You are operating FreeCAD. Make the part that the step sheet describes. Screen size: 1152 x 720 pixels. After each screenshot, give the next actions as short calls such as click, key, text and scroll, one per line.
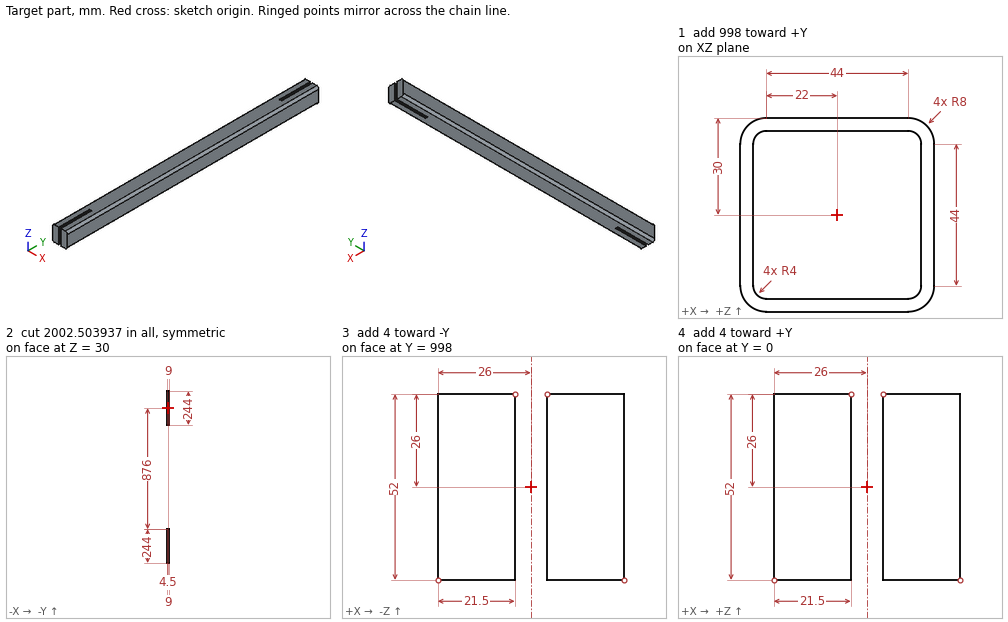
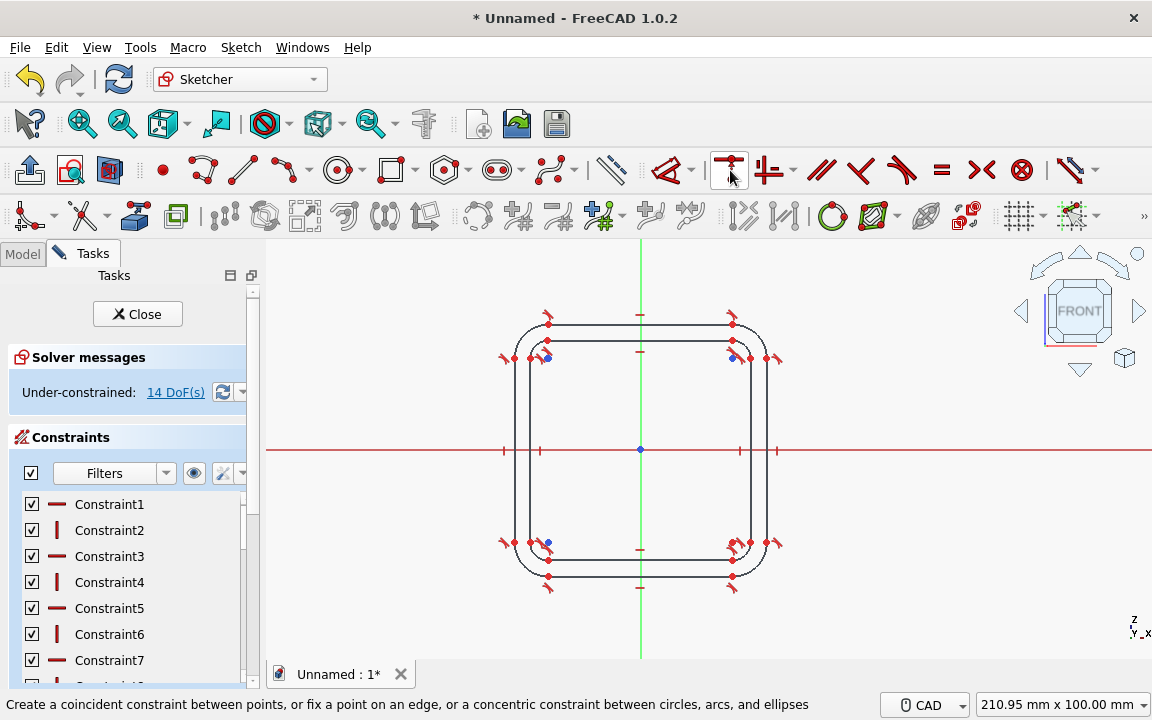
click(763, 343)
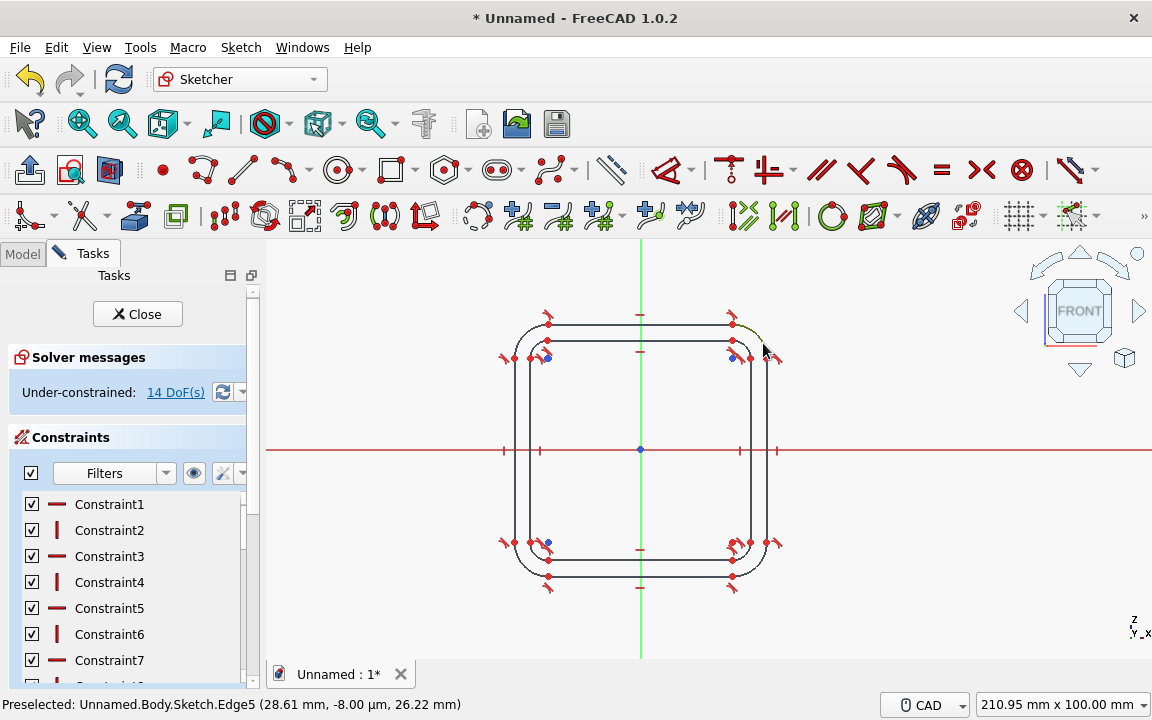
click(745, 346)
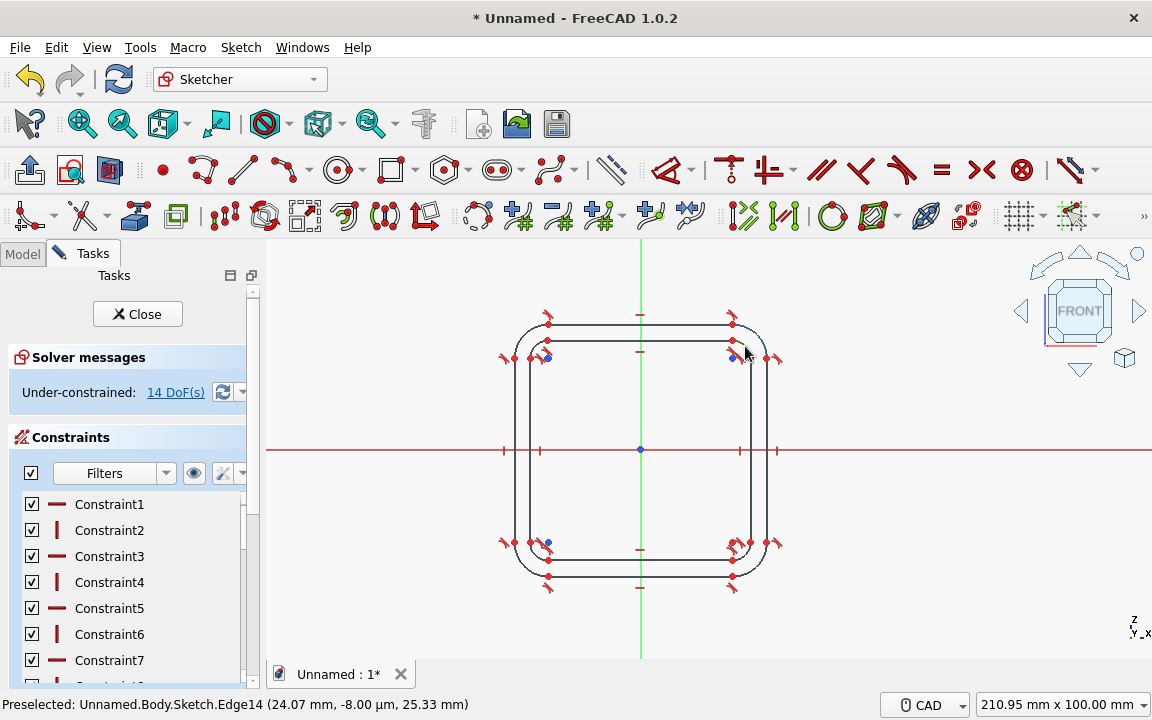
click(730, 170)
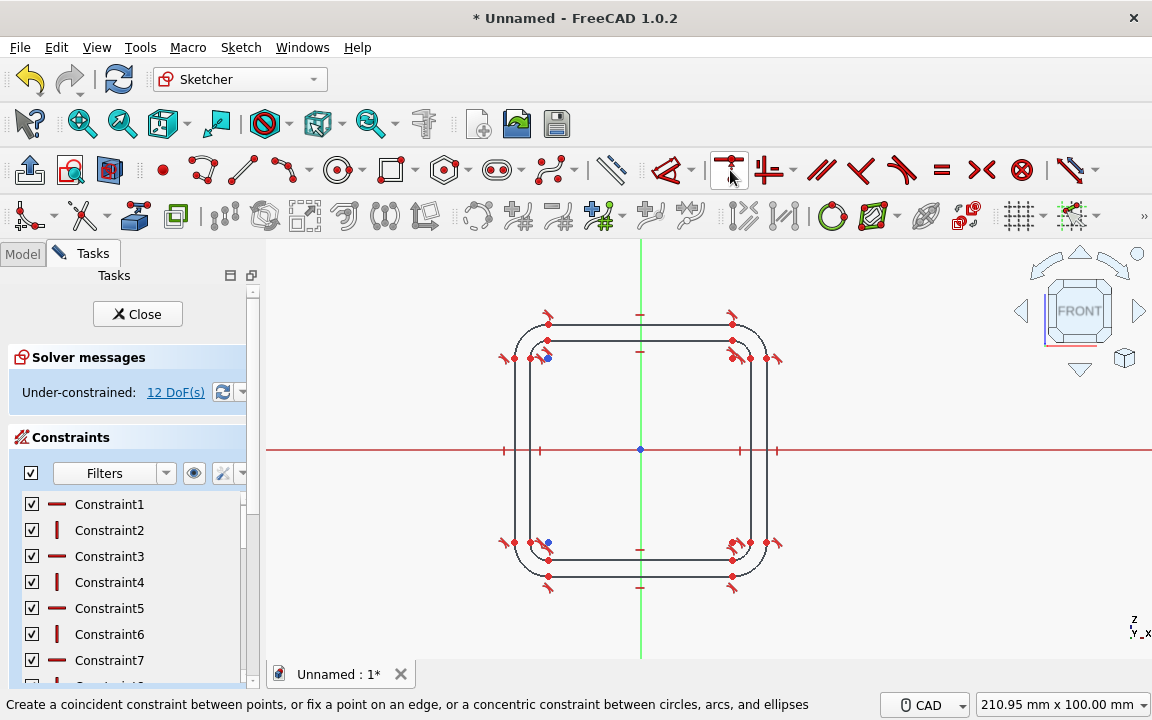
click(533, 328)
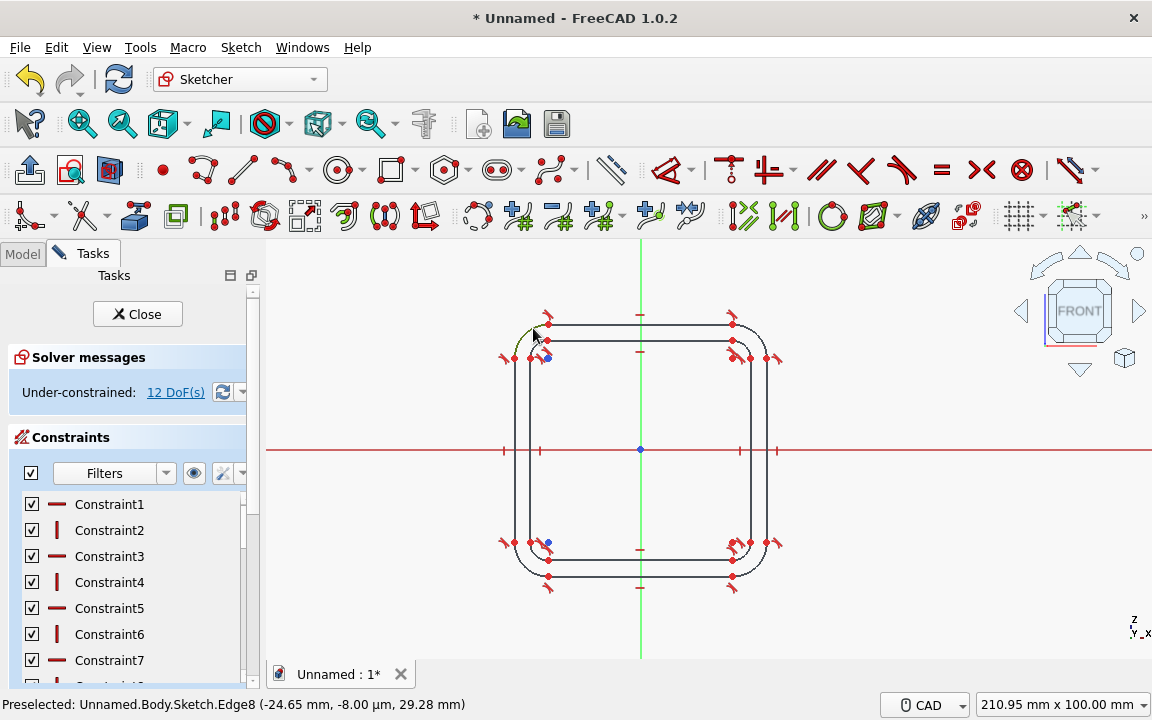
click(535, 346)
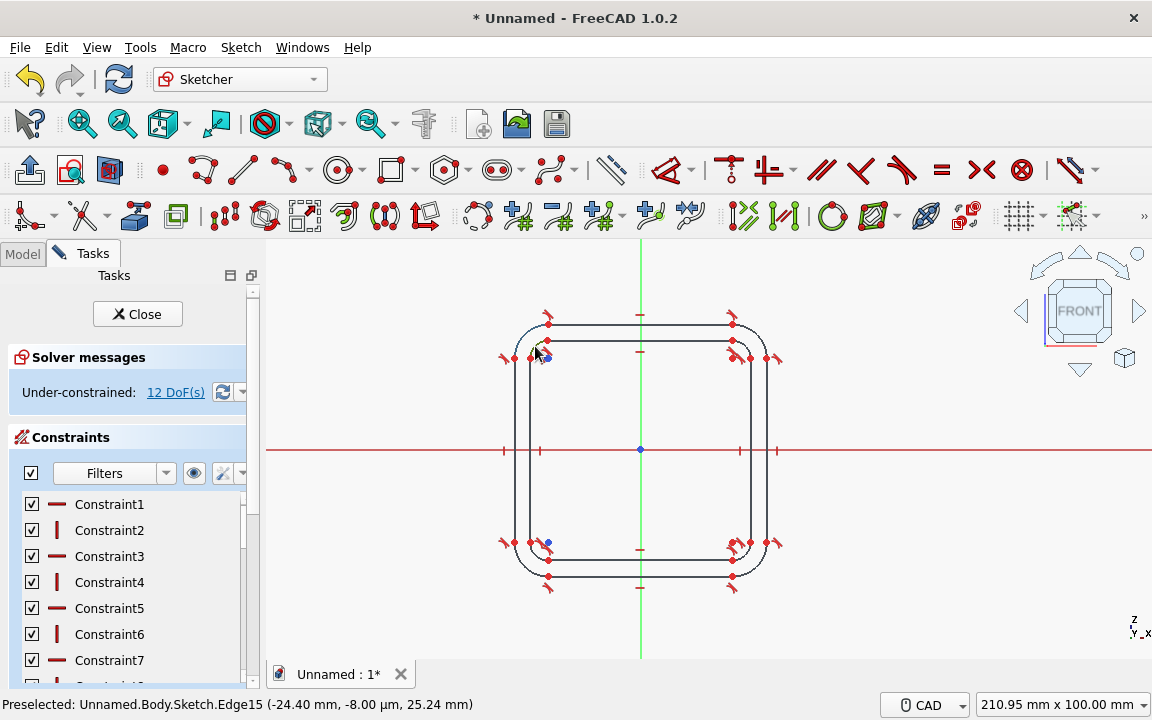
click(730, 170)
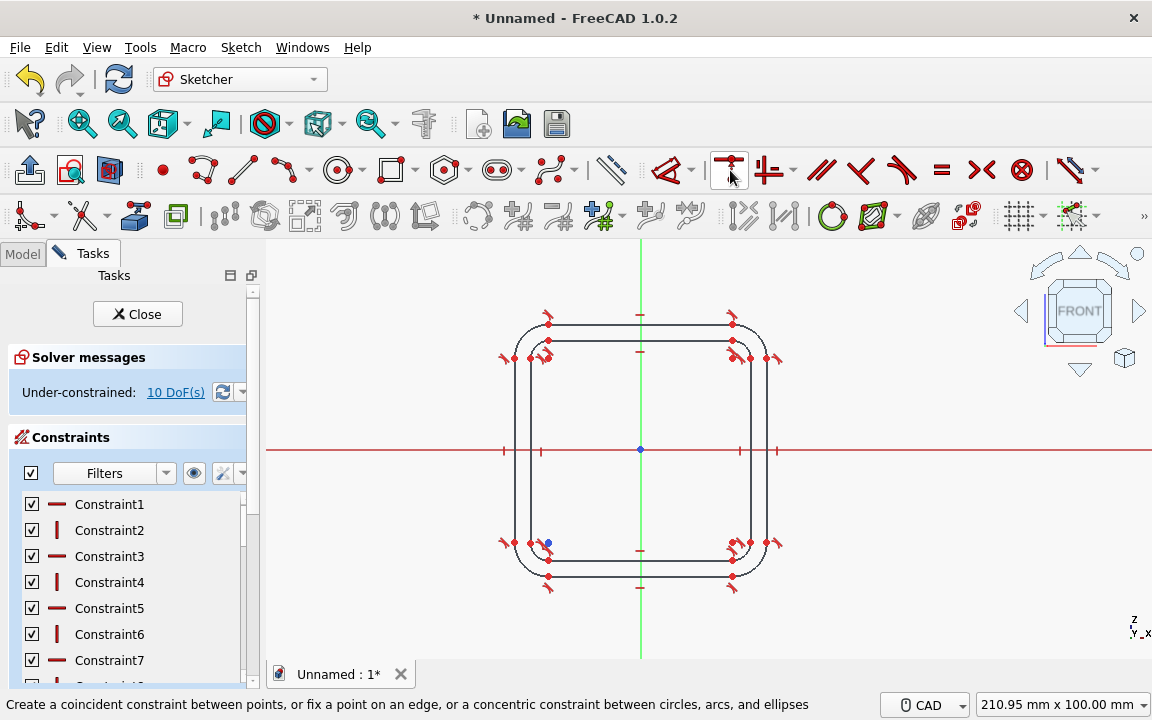
click(763, 343)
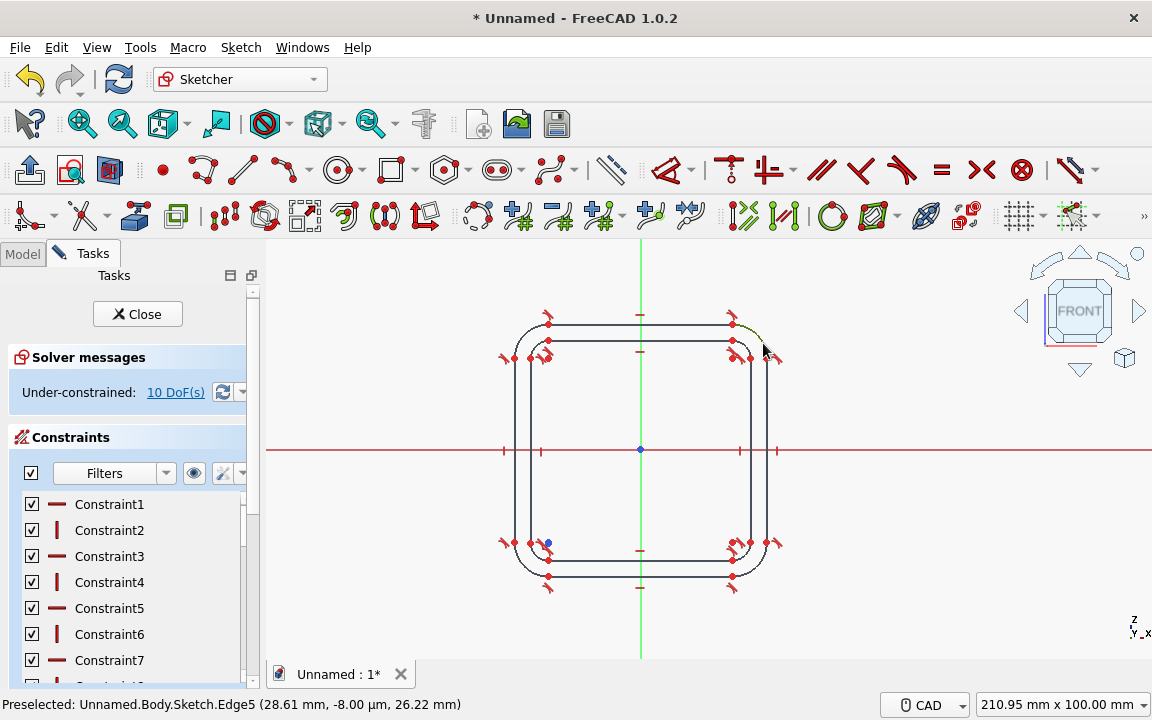
click(748, 573)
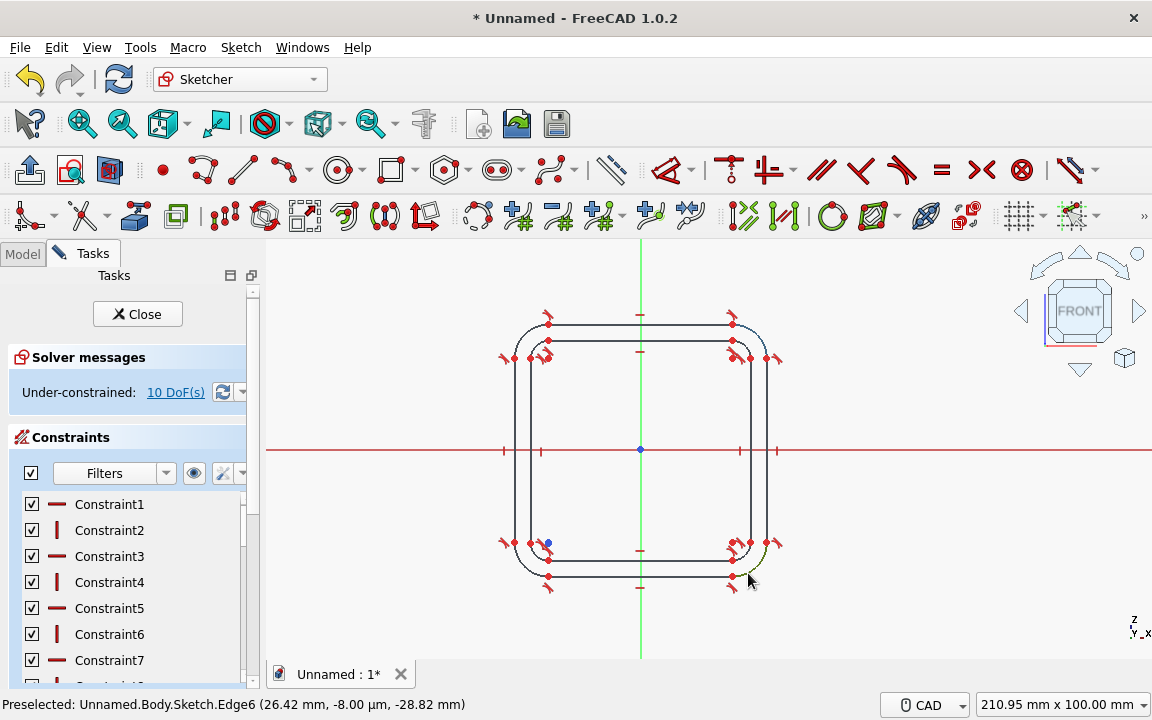
click(518, 558)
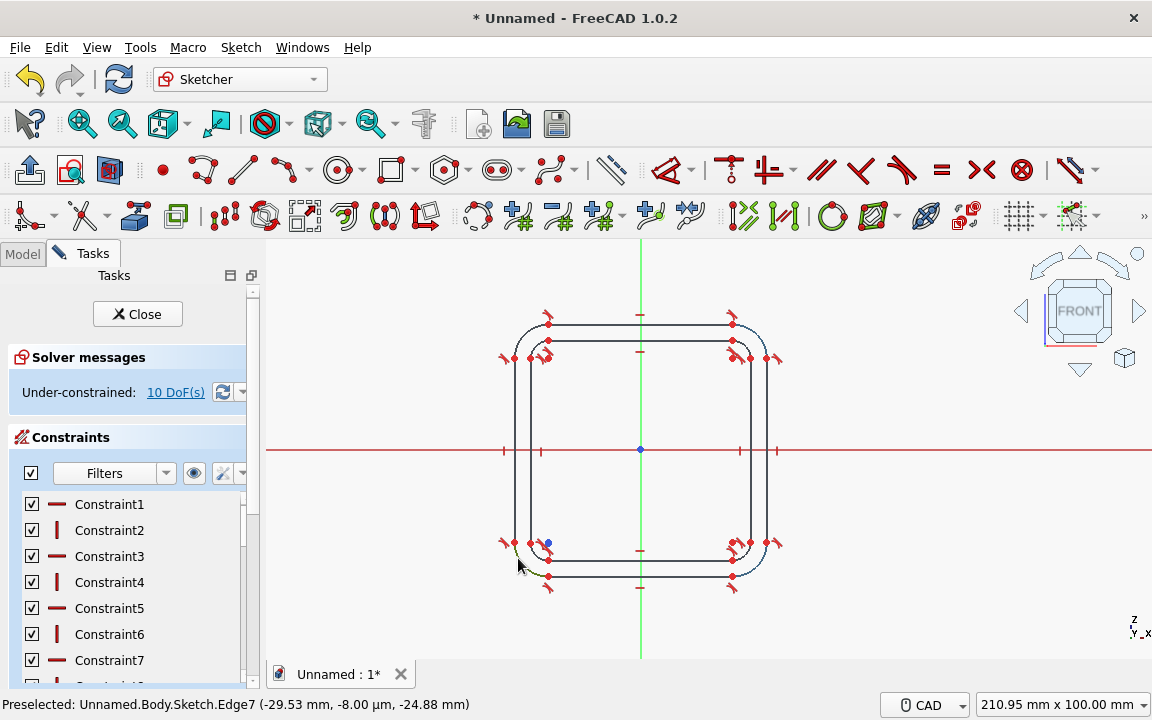
click(533, 328)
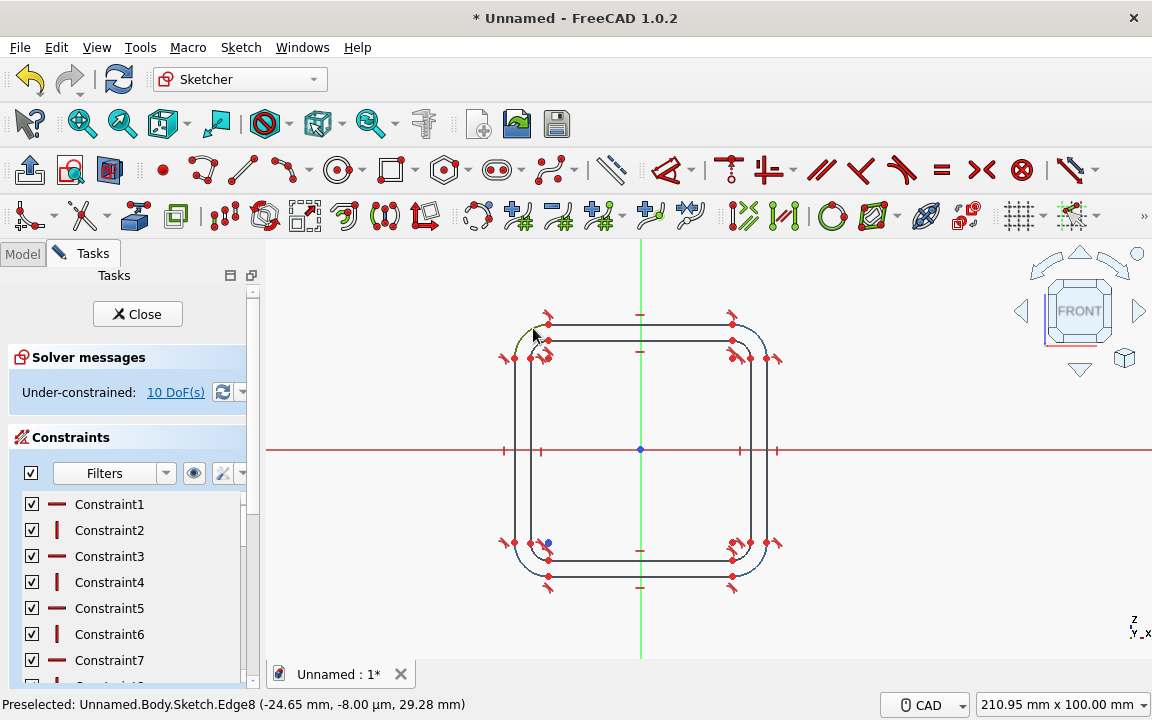
click(942, 170)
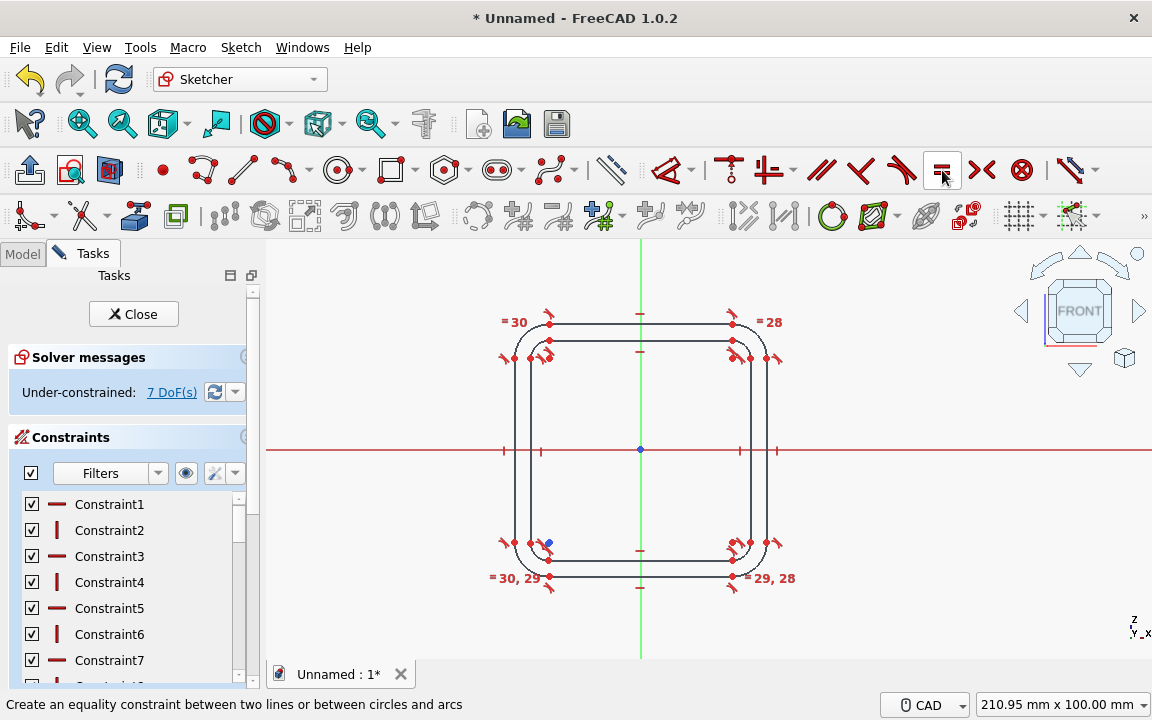
click(745, 555)